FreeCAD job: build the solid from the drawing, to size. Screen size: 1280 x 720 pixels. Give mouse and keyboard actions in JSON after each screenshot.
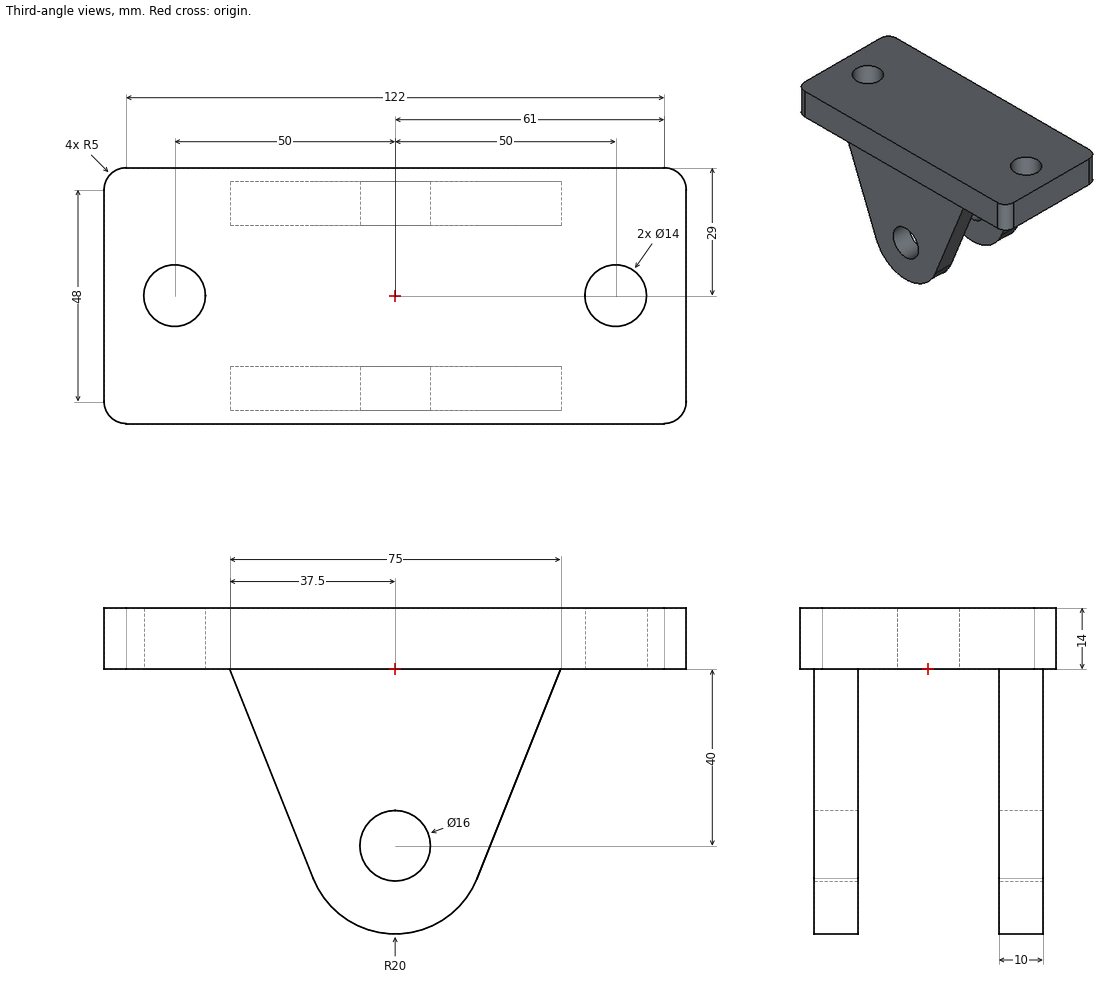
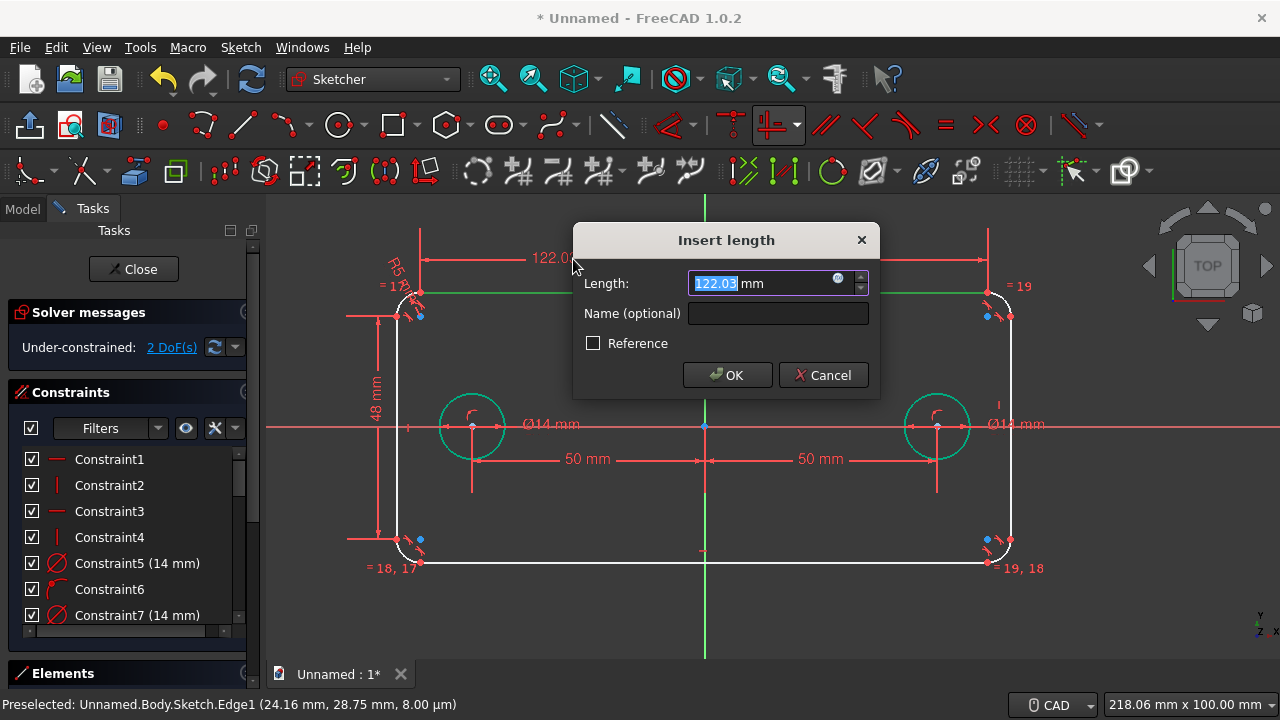
{"action": "type", "text": "122"}
{"action": "key", "text": "Return"}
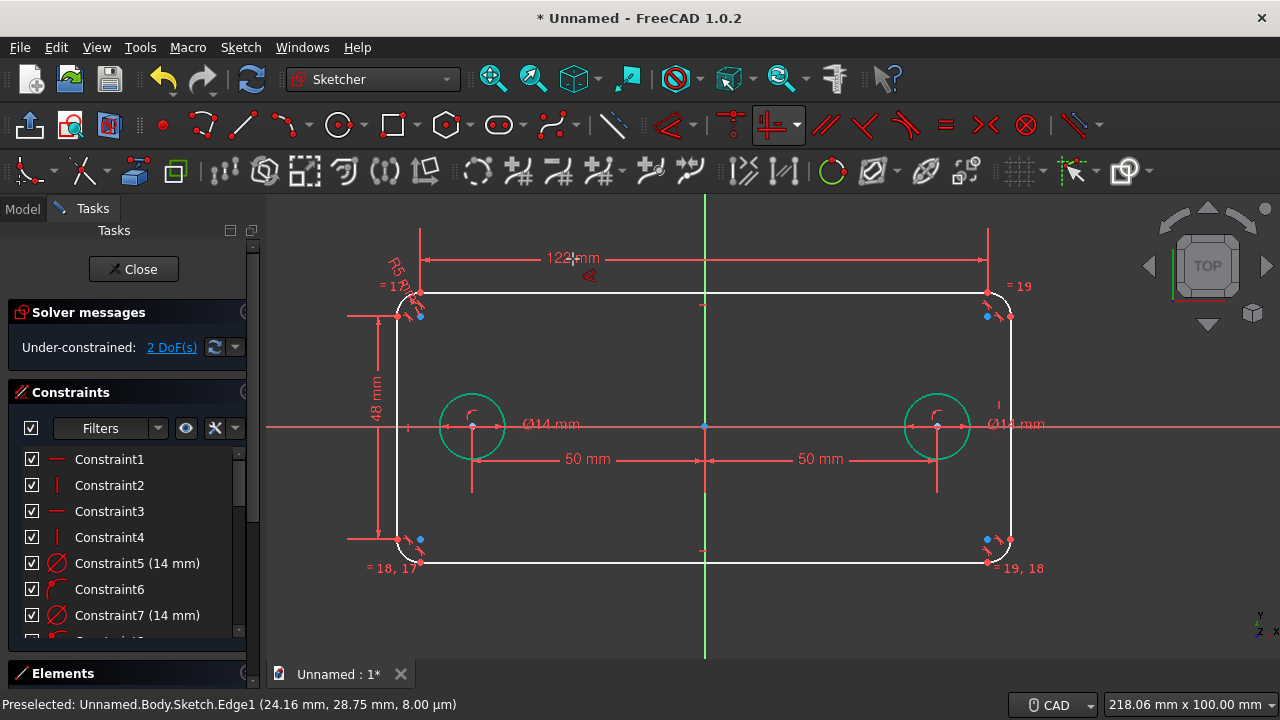
{"action": "left_click", "coordinate": [988, 293]}
{"action": "left_click", "coordinate": [846, 259]}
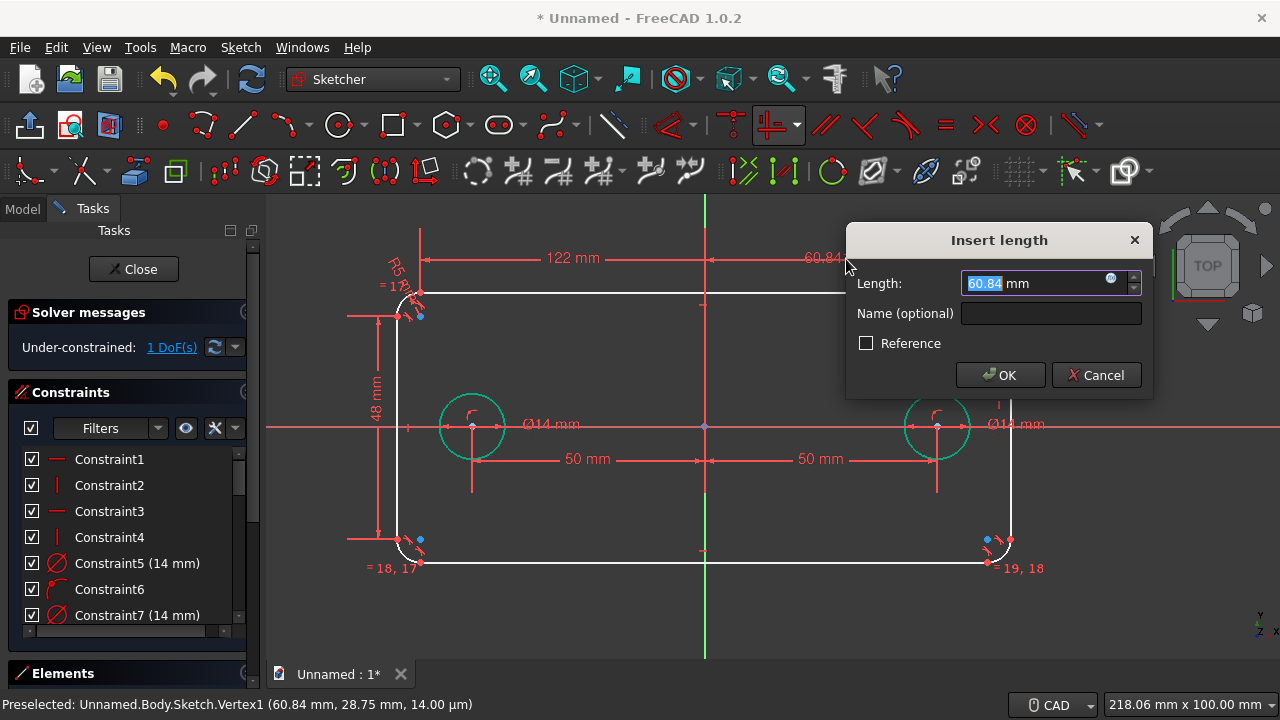
{"action": "type", "text": "61"}
{"action": "key", "text": "Return"}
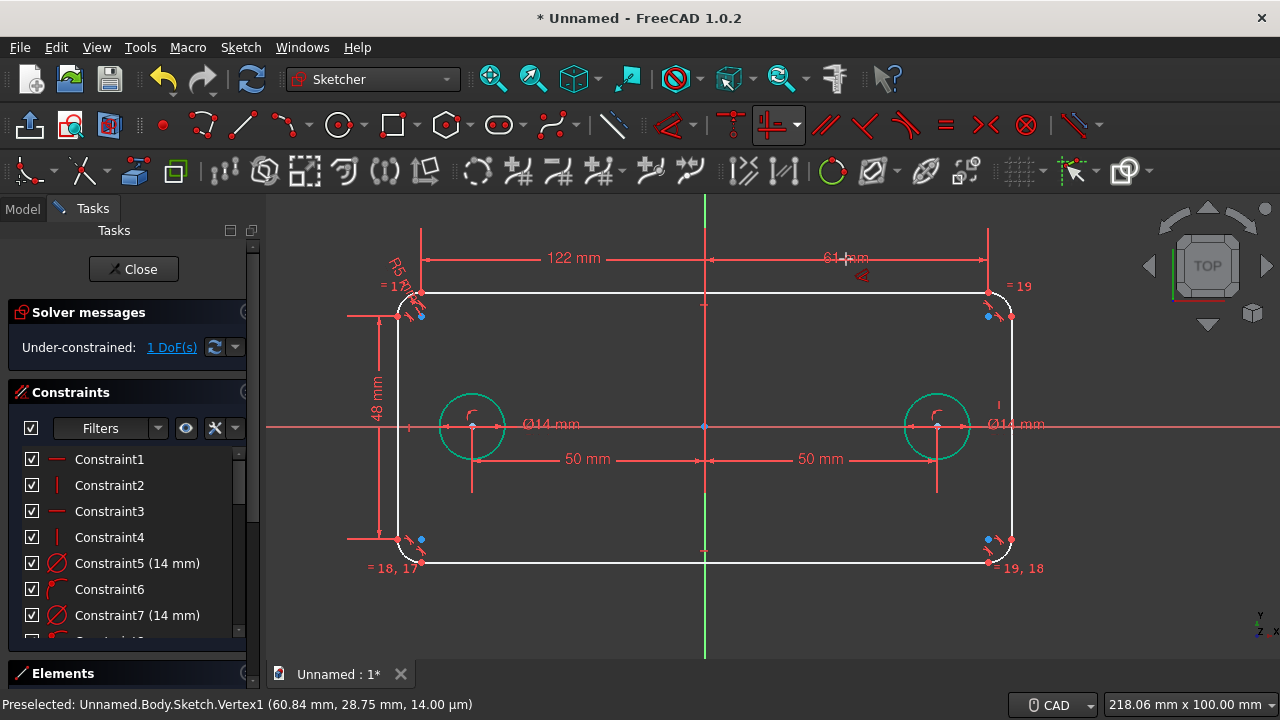
{"action": "left_click", "coordinate": [988, 293]}
{"action": "left_click", "coordinate": [671, 360]}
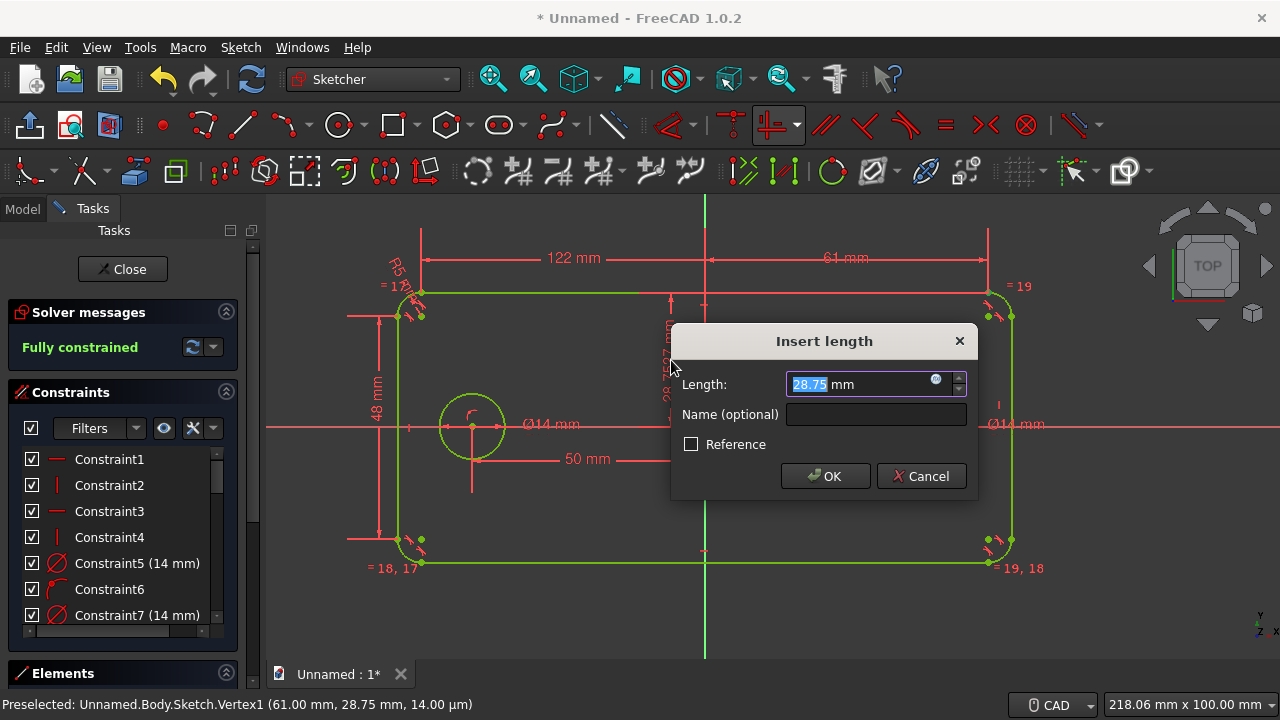
{"action": "type", "text": "29"}
{"action": "key", "text": "Return"}
{"action": "key", "text": "Escape"}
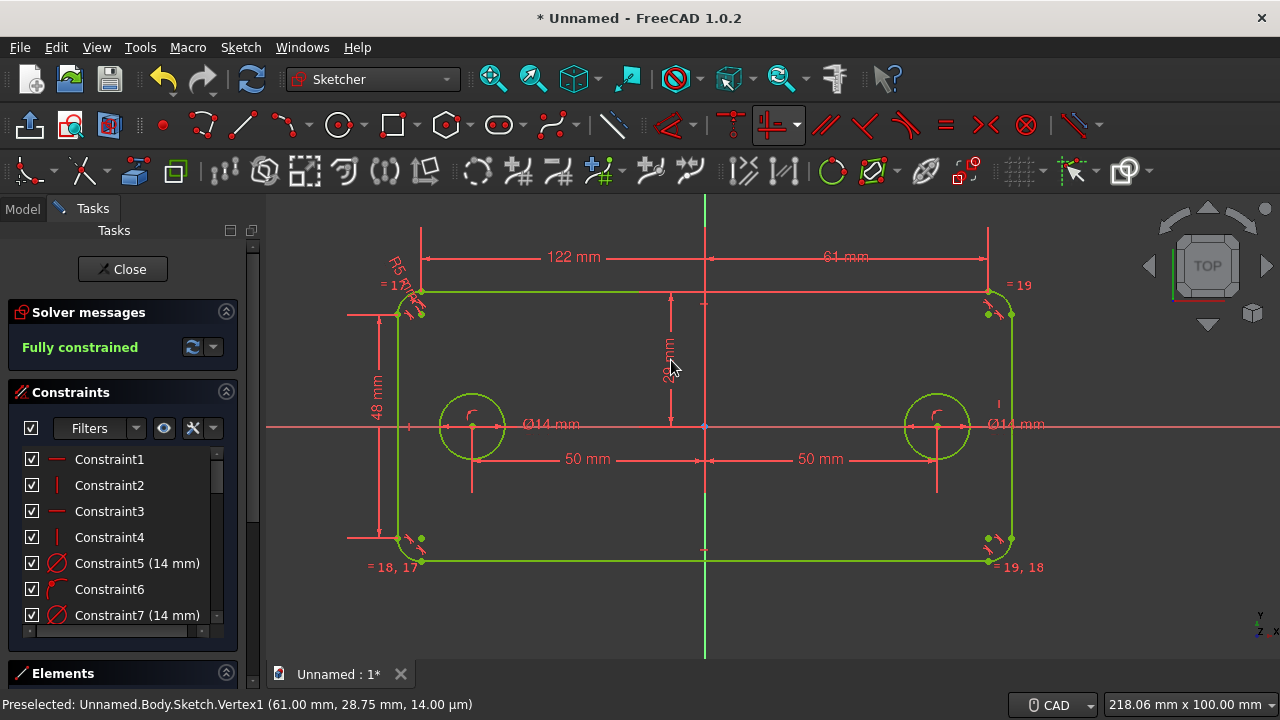
{"action": "left_click", "coordinate": [123, 269]}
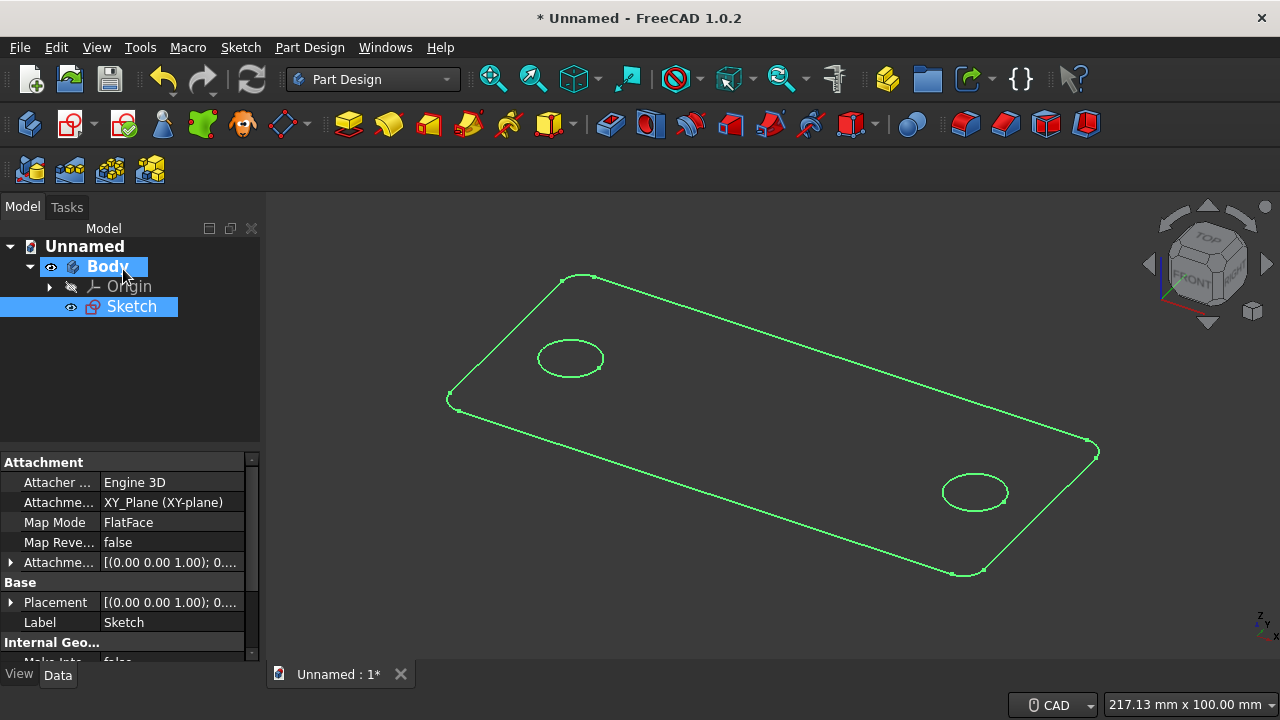
{"action": "left_click", "coordinate": [350, 124]}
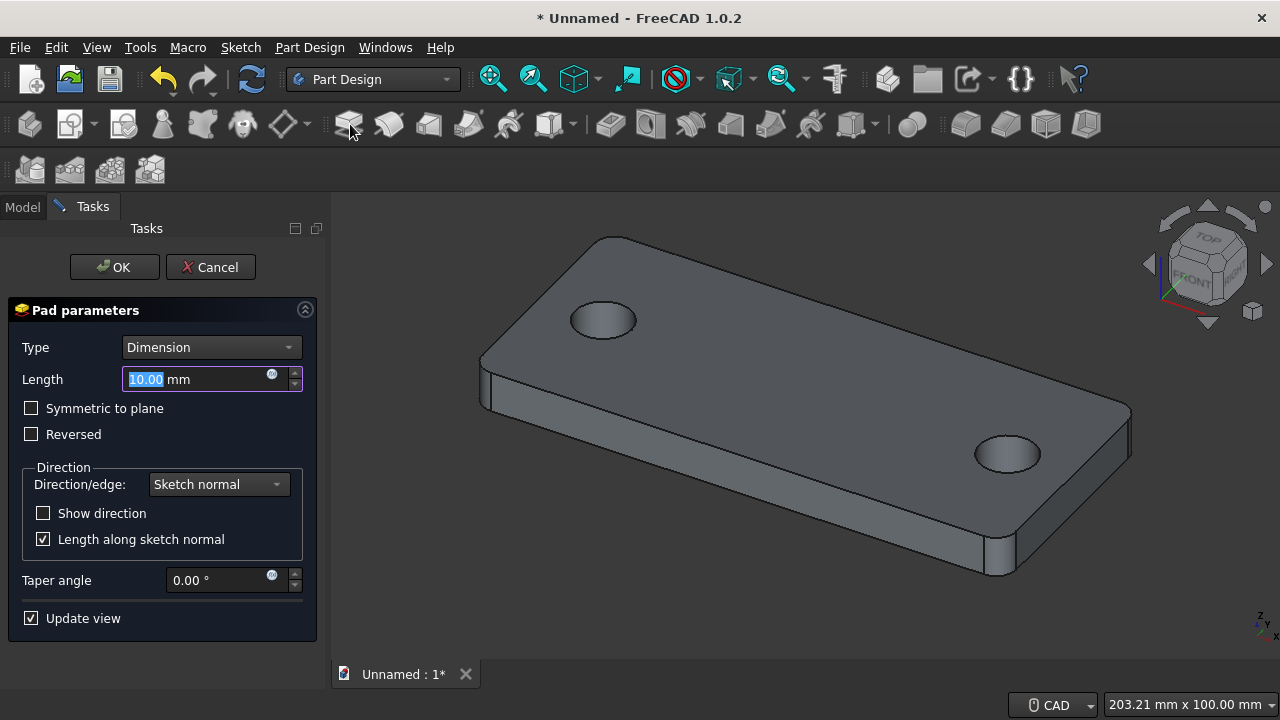
{"action": "type", "text": "14"}
{"action": "key", "text": "Tab"}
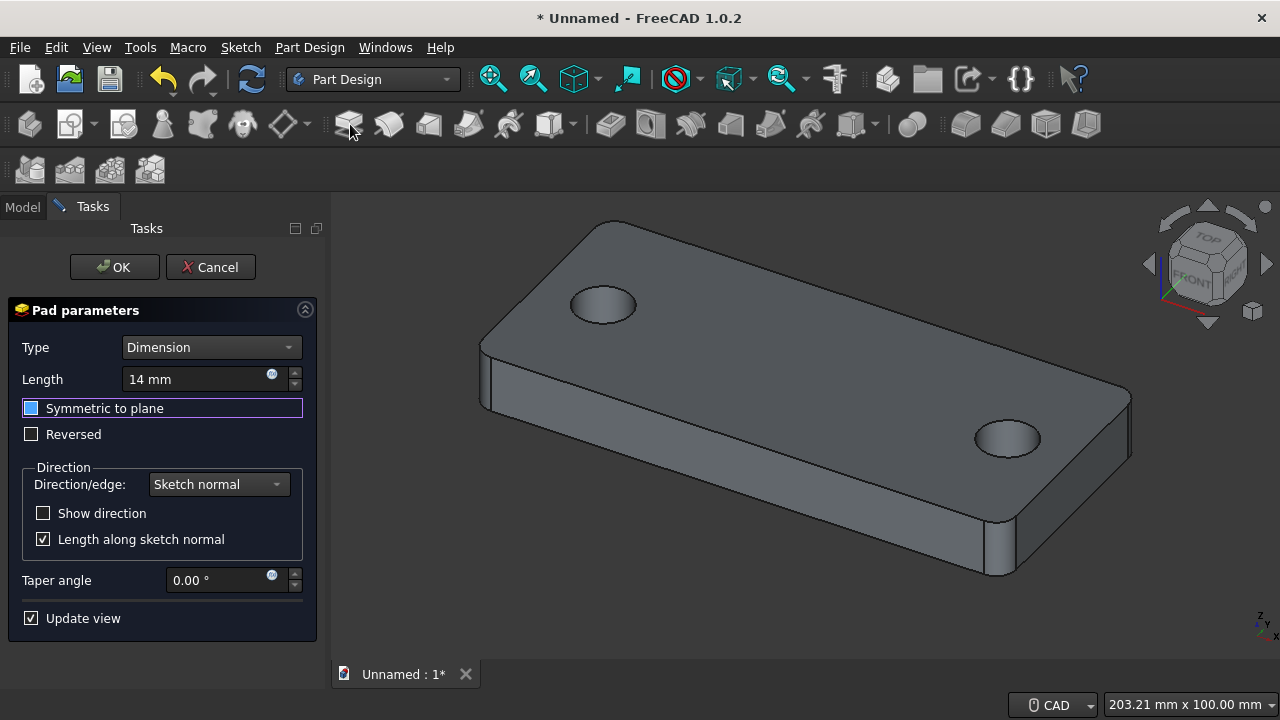
{"action": "left_click", "coordinate": [115, 267]}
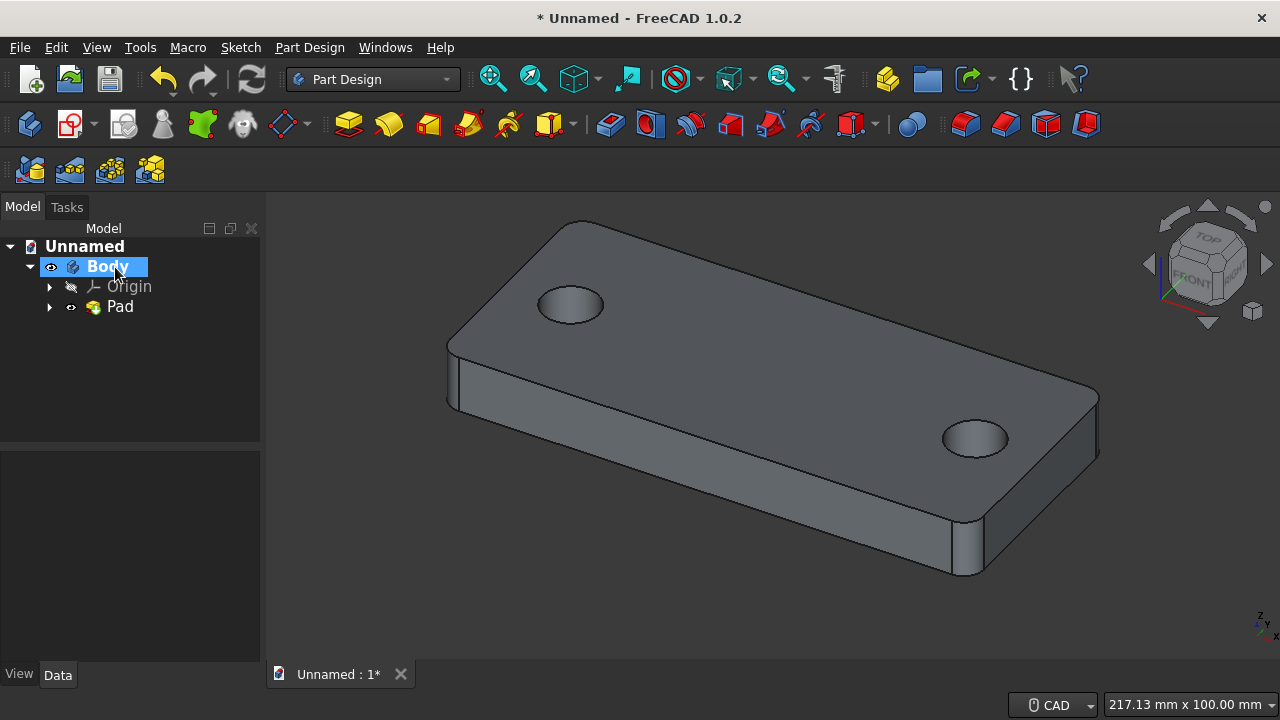
{"action": "left_click", "coordinate": [50, 287]}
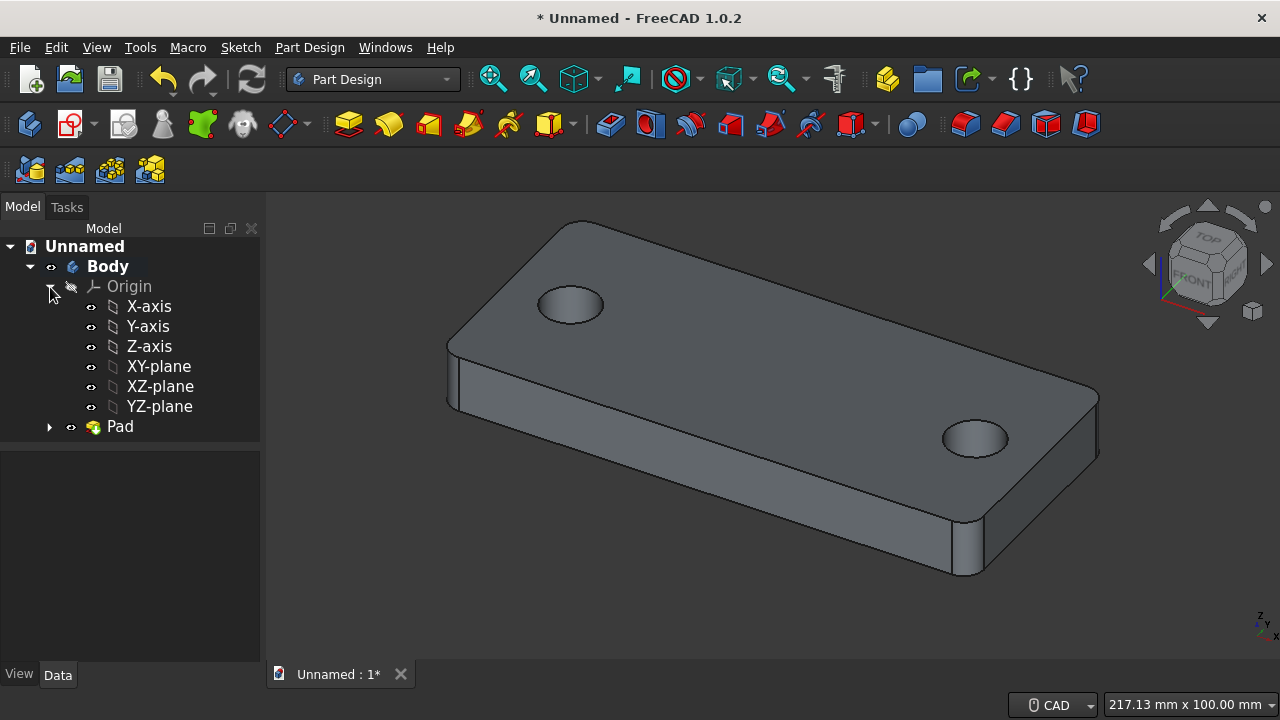
{"action": "left_click", "coordinate": [136, 387]}